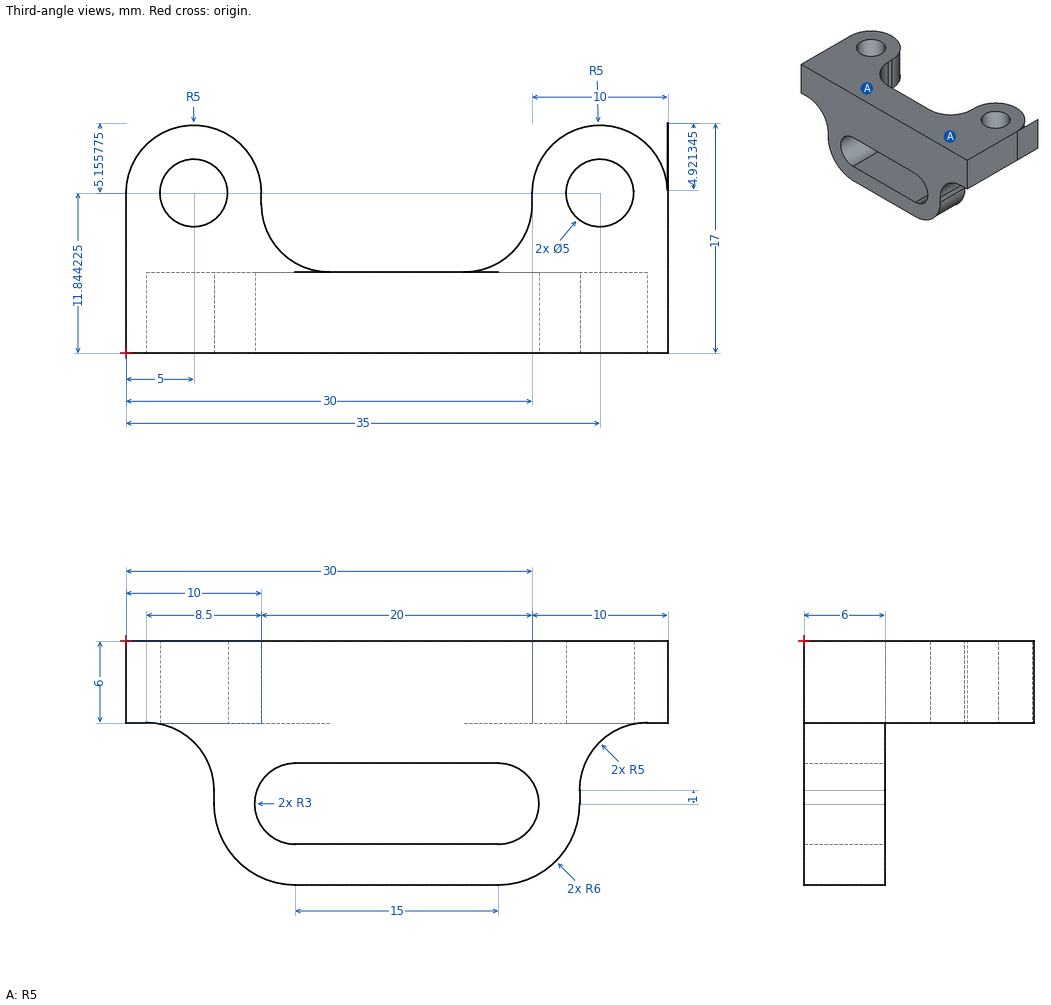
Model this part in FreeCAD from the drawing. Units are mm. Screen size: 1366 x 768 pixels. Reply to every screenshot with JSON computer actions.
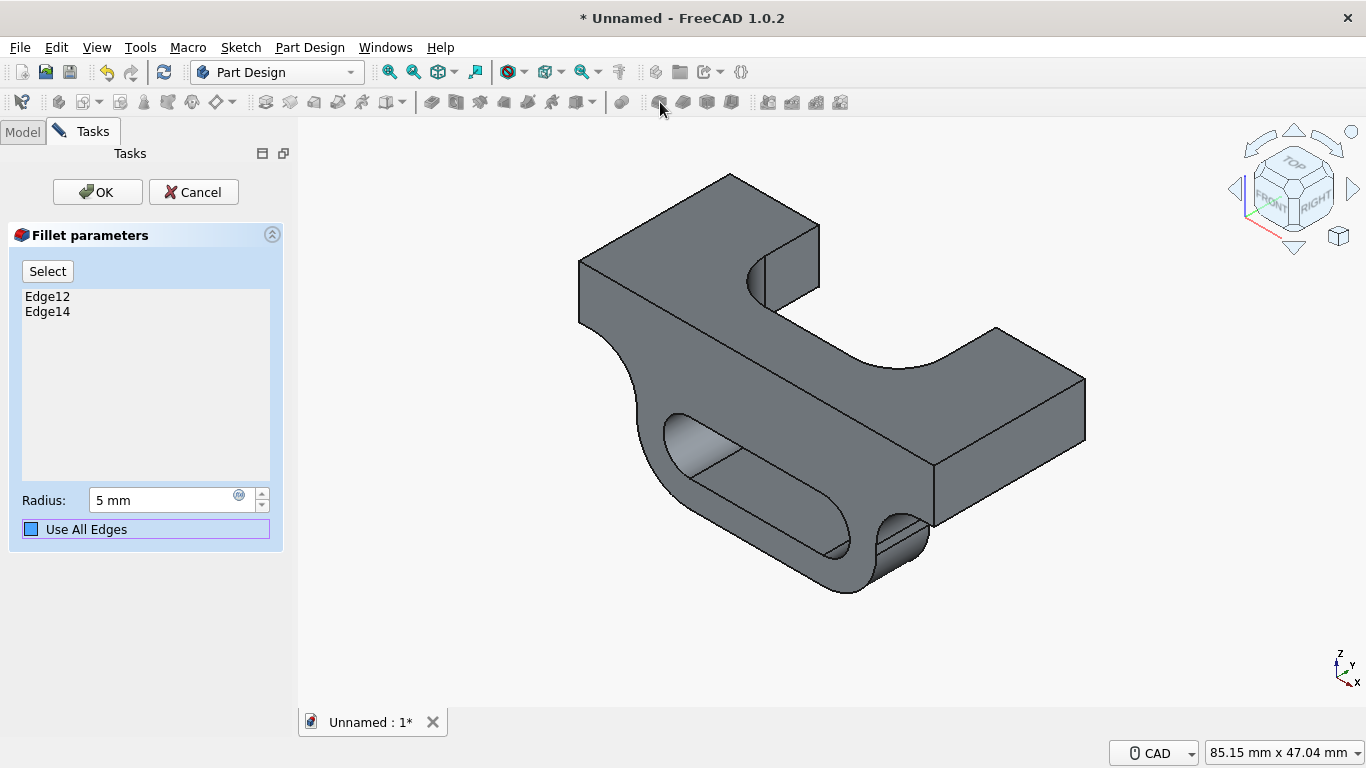
{"action": "left_click", "coordinate": [98, 192]}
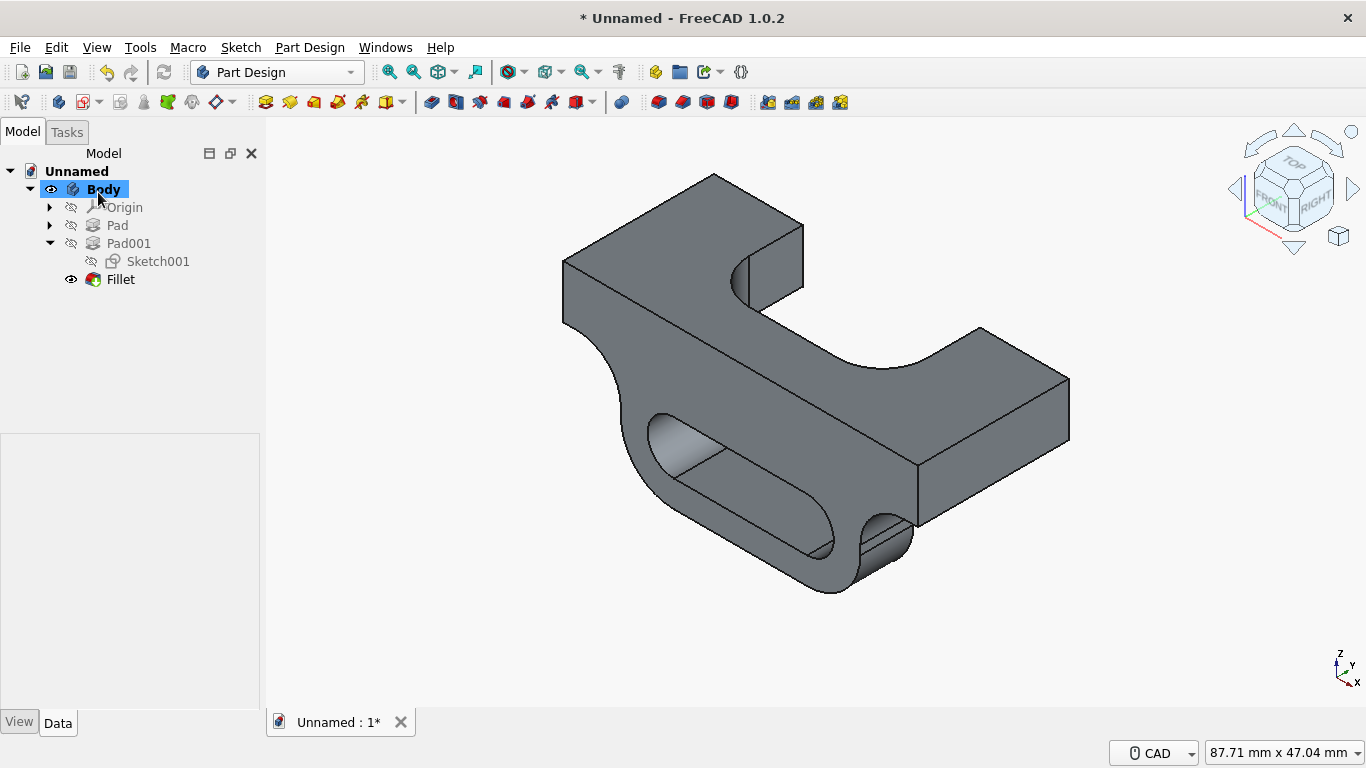
{"action": "key", "text": "5"}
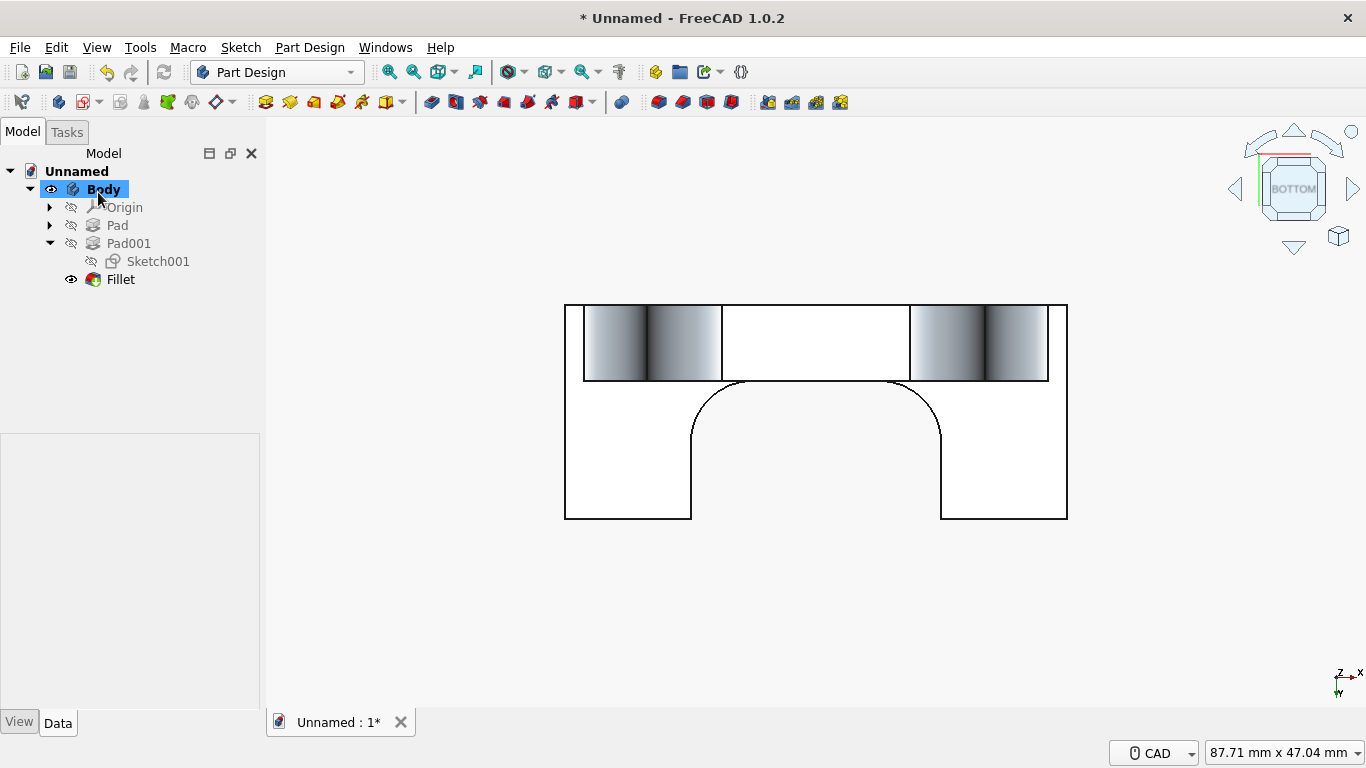
{"action": "left_click", "coordinate": [632, 441]}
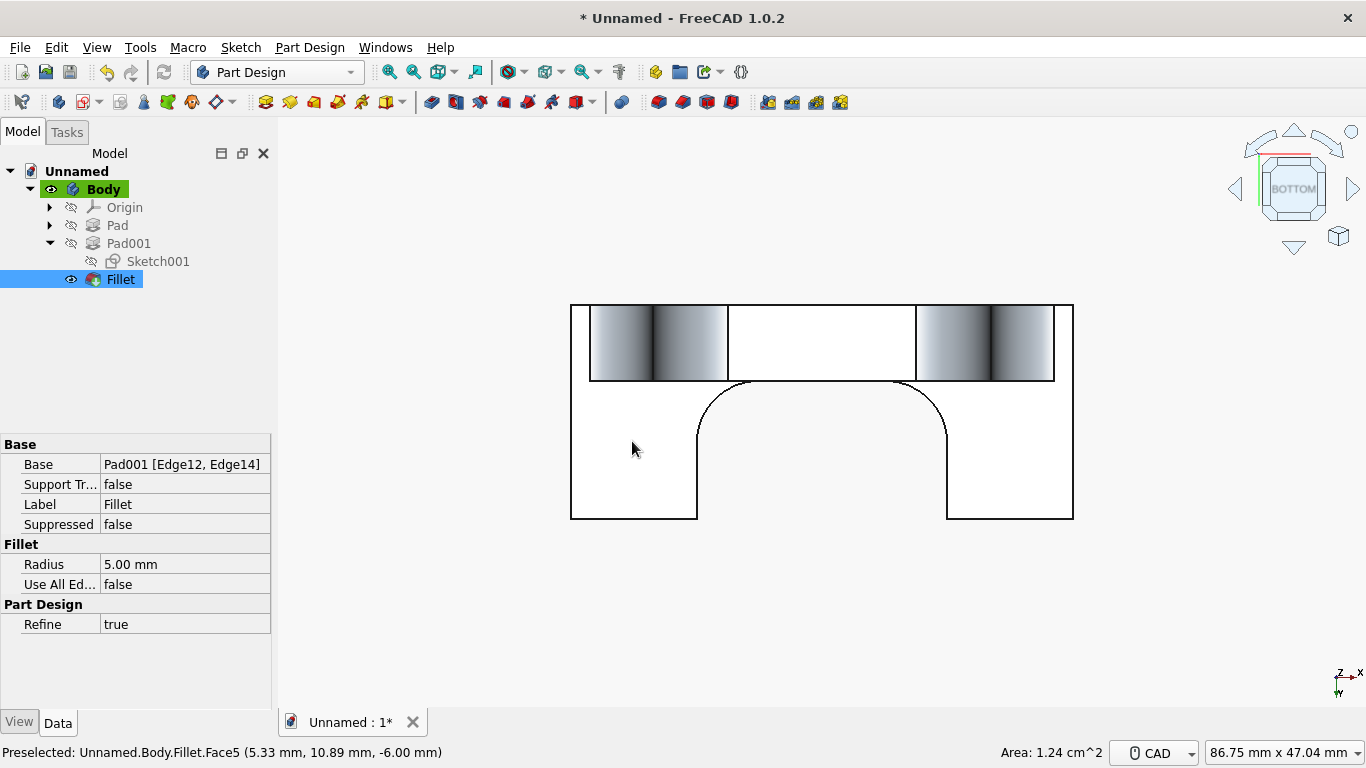
{"action": "left_click", "coordinate": [84, 102]}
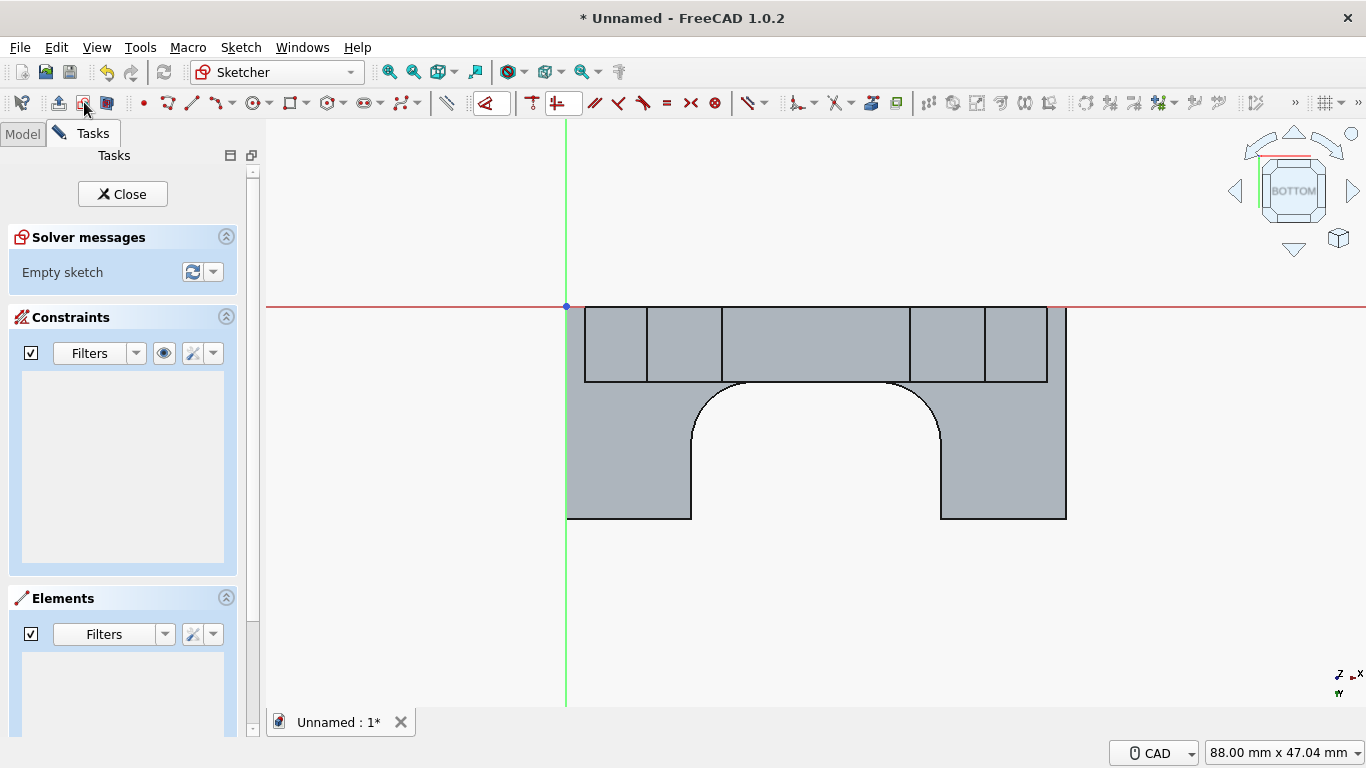
{"action": "scroll", "coordinate": [908, 363], "scroll_direction": "up", "scroll_amount": 2}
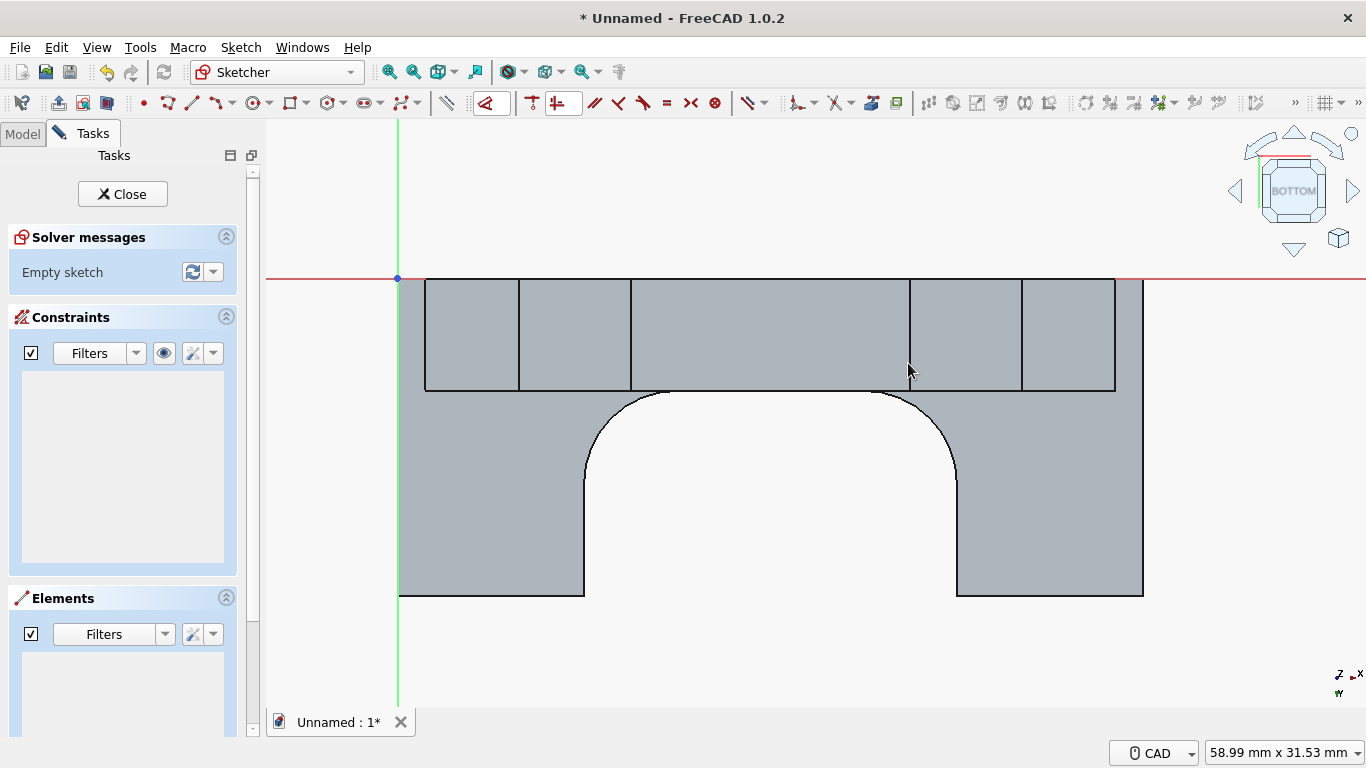
{"action": "key", "text": "g c"}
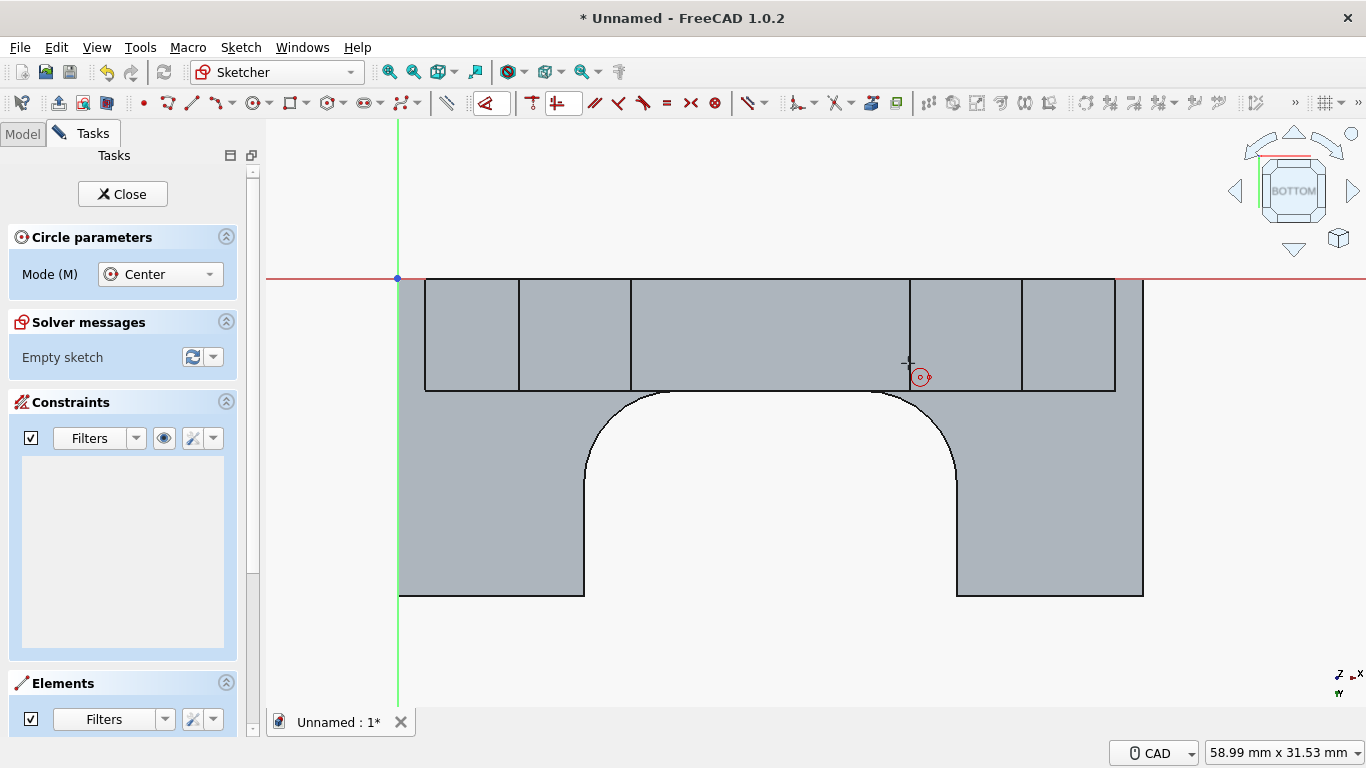
{"action": "left_click", "coordinate": [1050, 500]}
{"action": "mouse_move", "coordinate": [1083, 467]}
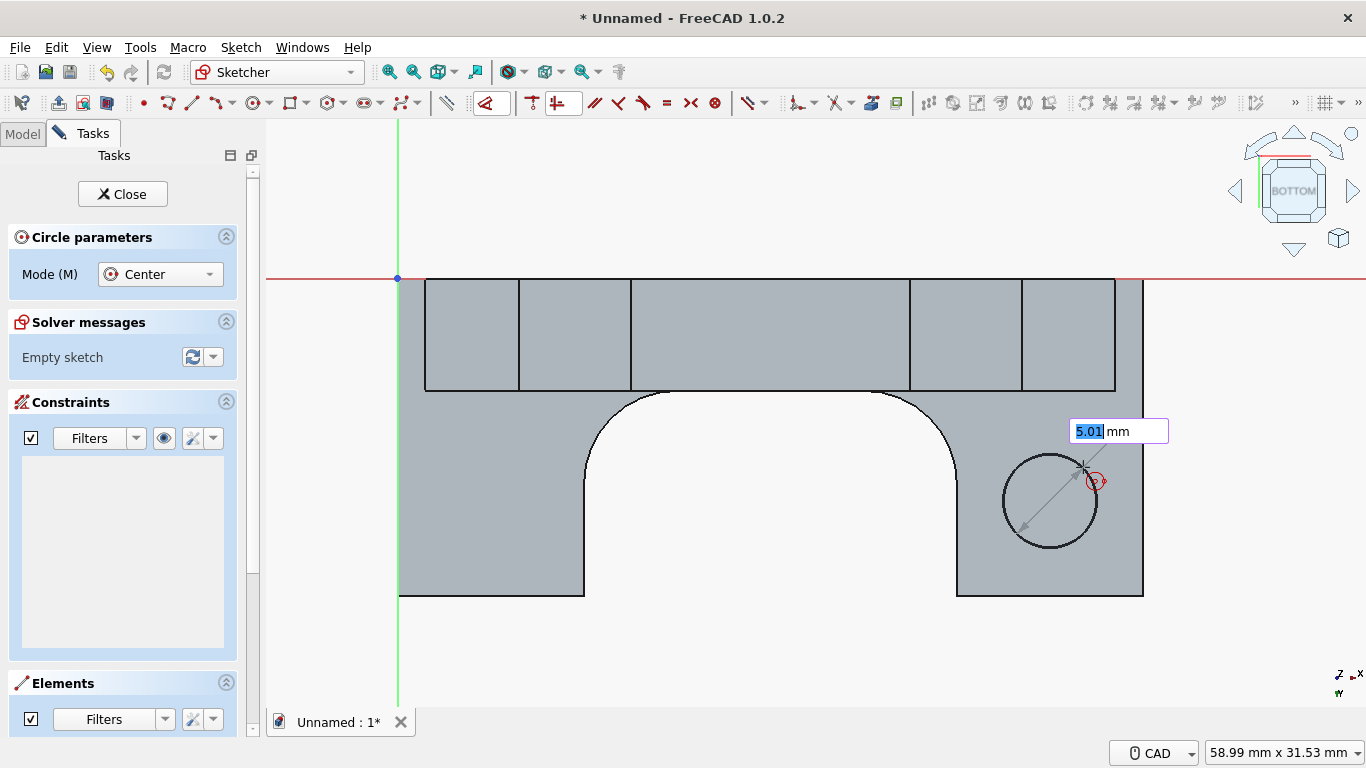
{"action": "type", "text": "5"}
{"action": "key", "text": "Return"}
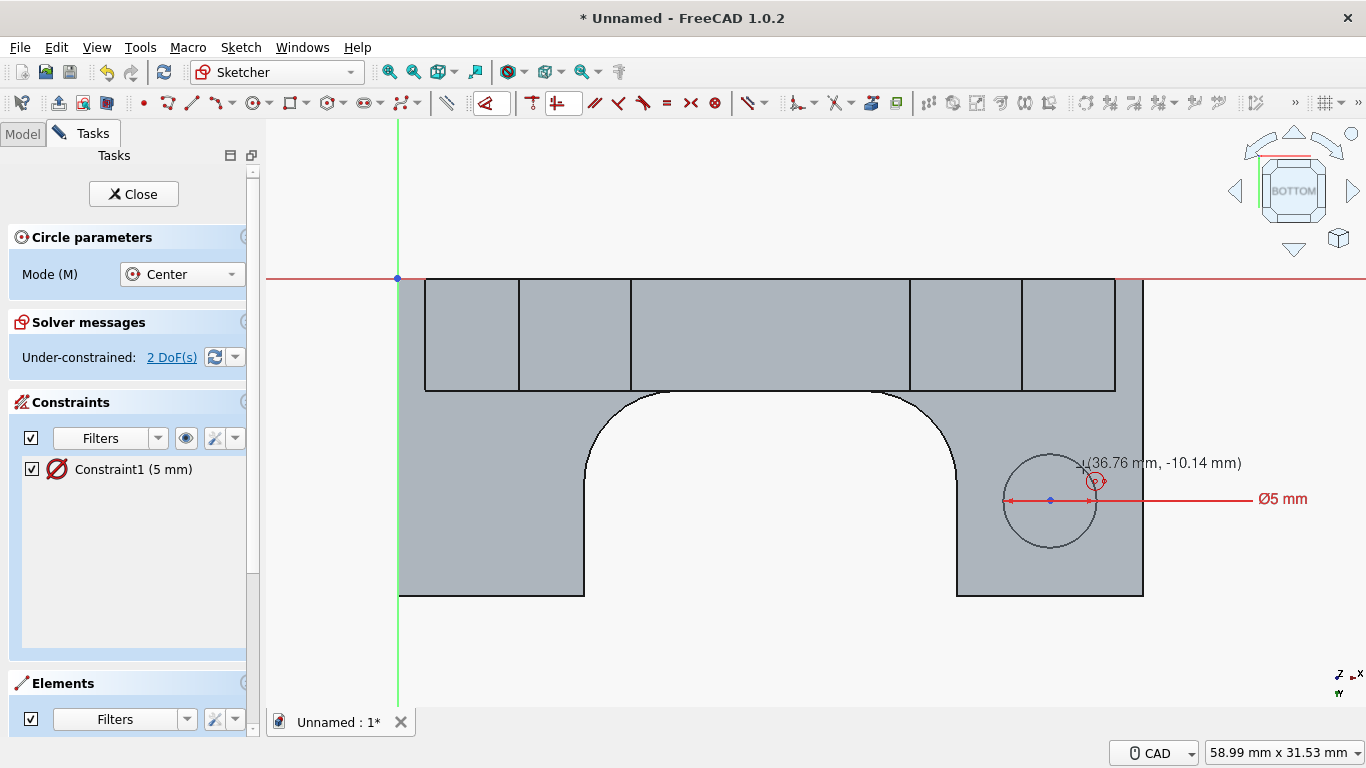
{"action": "left_click", "coordinate": [491, 500]}
{"action": "mouse_move", "coordinate": [524, 467]}